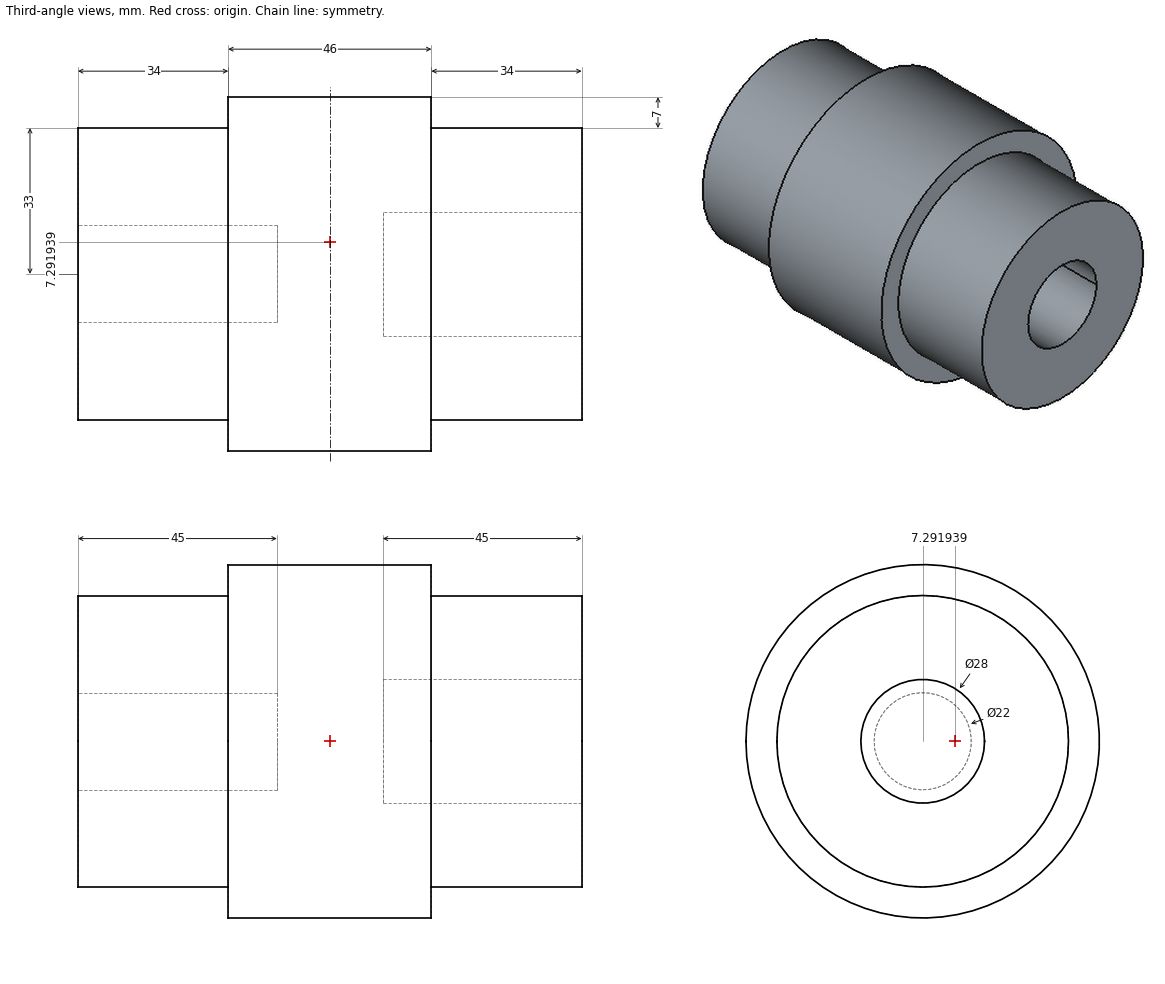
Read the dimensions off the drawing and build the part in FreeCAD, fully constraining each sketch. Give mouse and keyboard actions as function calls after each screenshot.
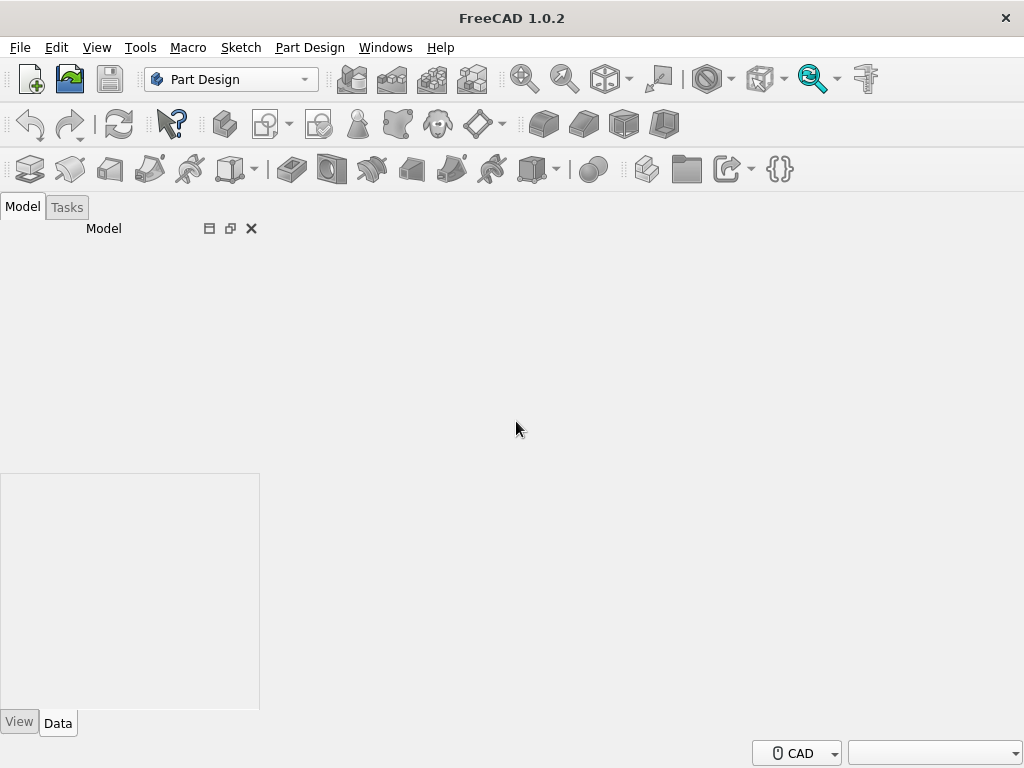
click(30, 80)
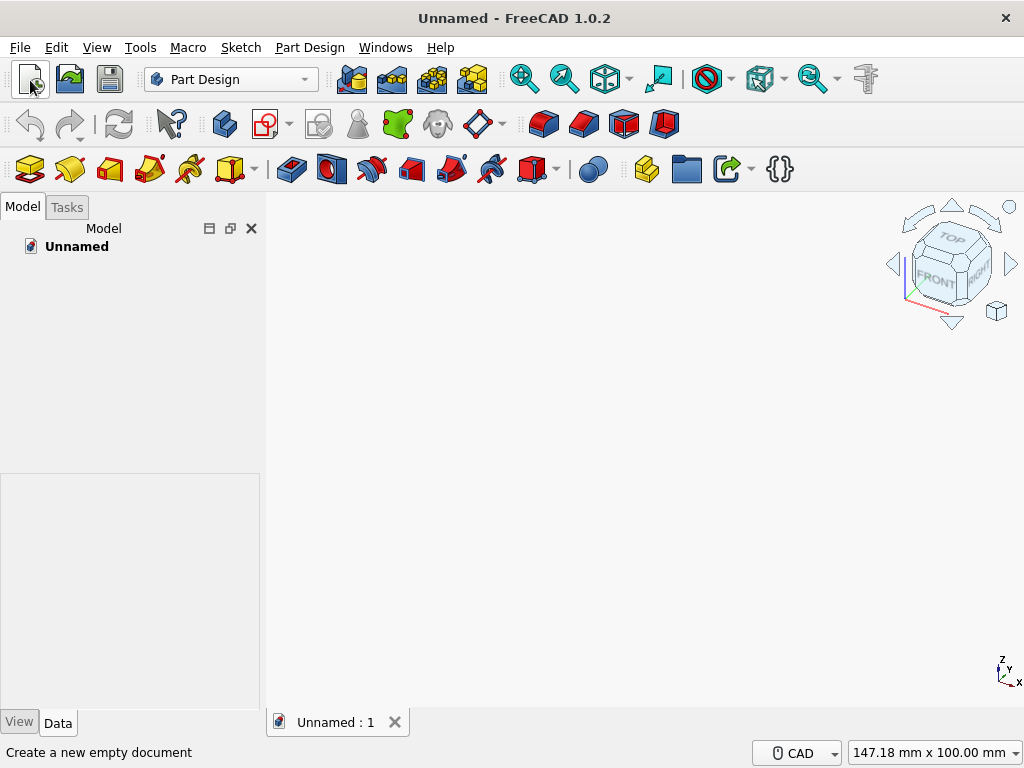
click(266, 124)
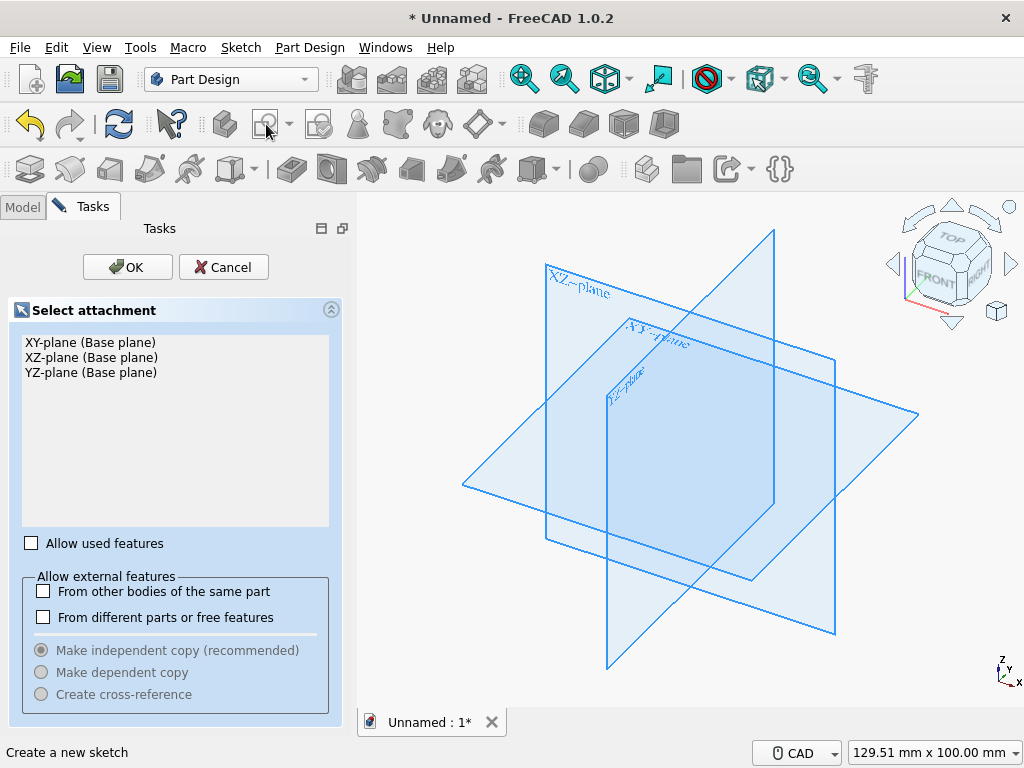
click(82, 342)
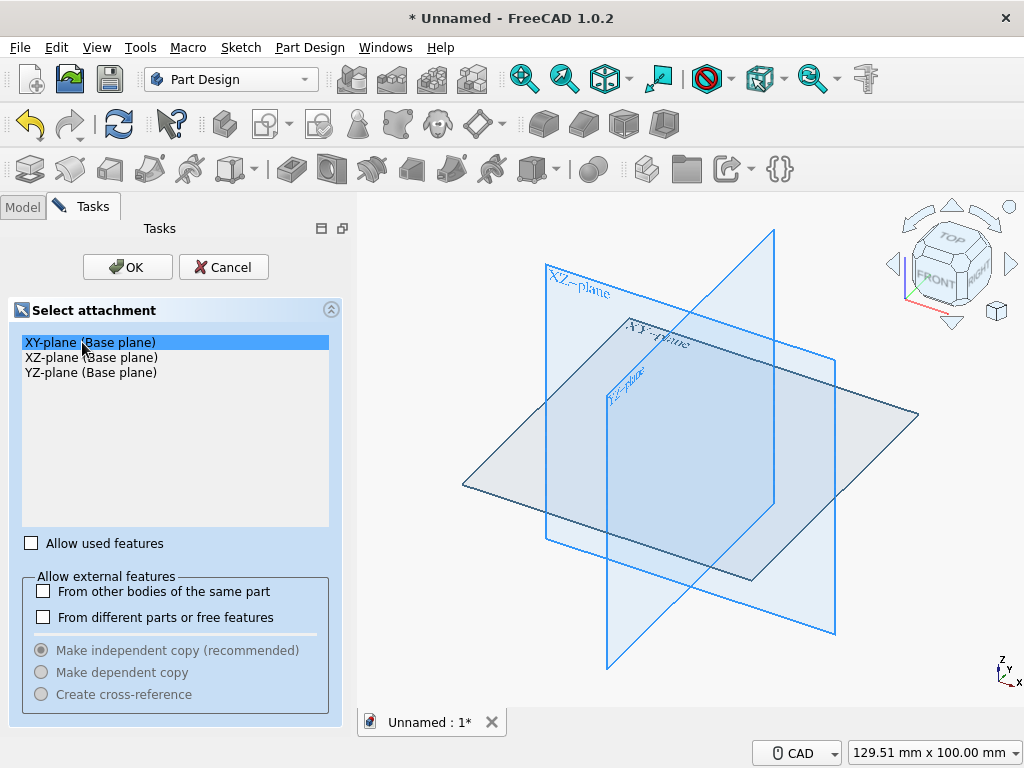
click(128, 267)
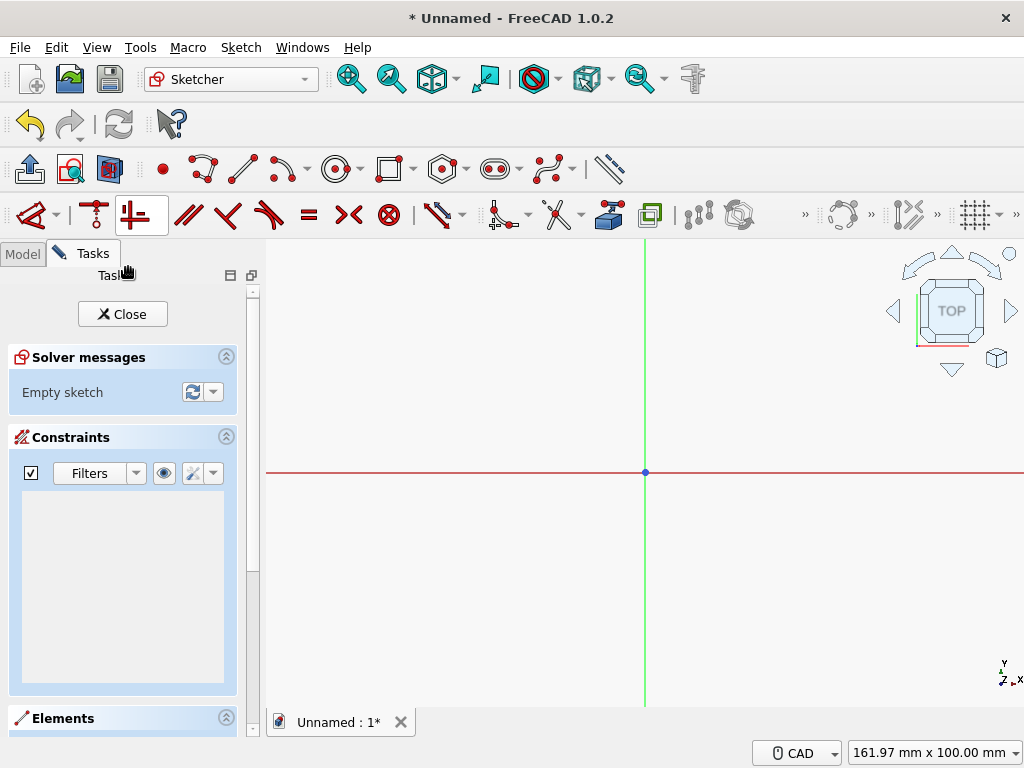
scroll(363, 545, down, 3)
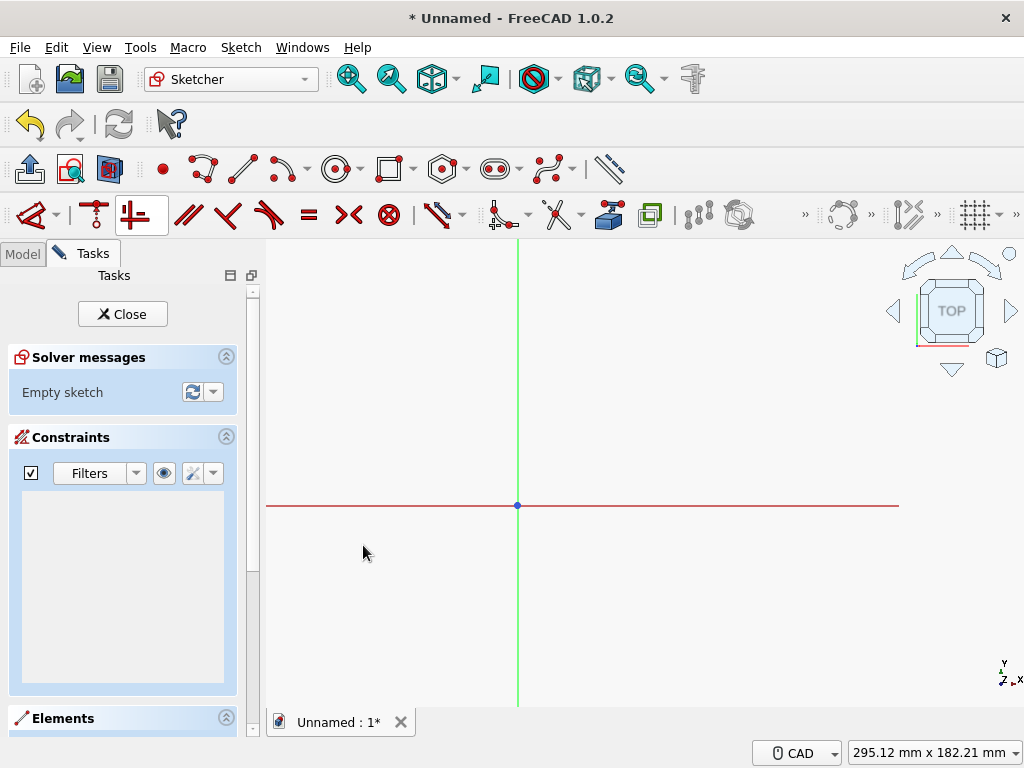
click(204, 170)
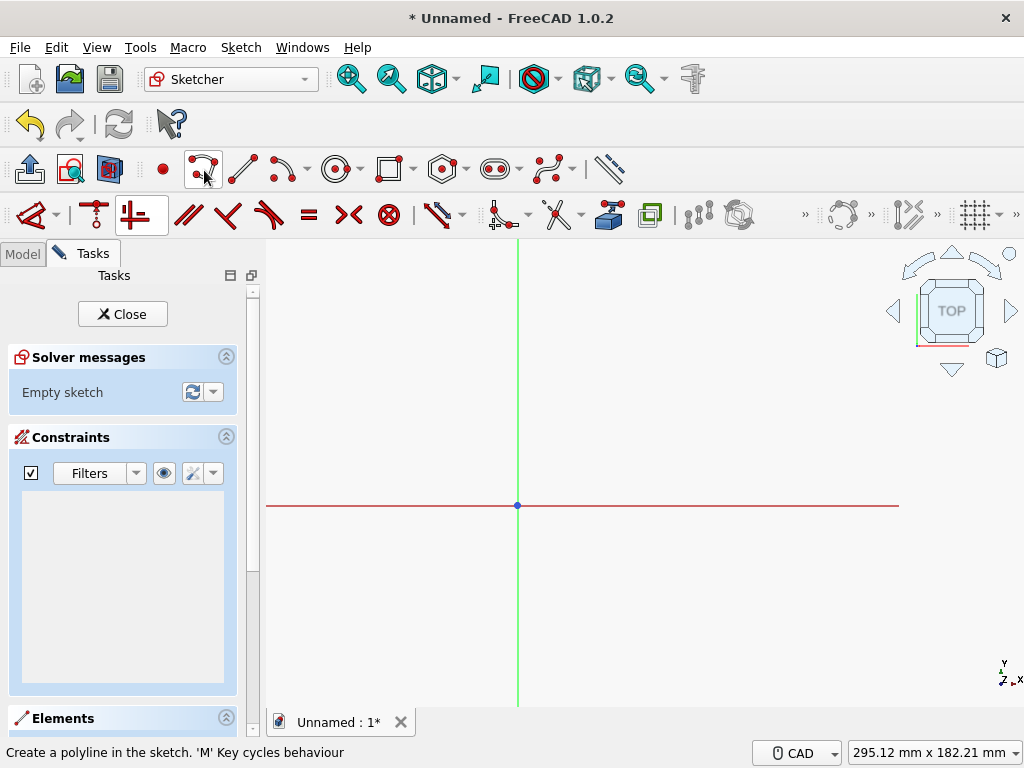
click(577, 440)
click(577, 422)
click(459, 422)
click(459, 440)
click(371, 440)
click(371, 525)
click(664, 525)
click(664, 440)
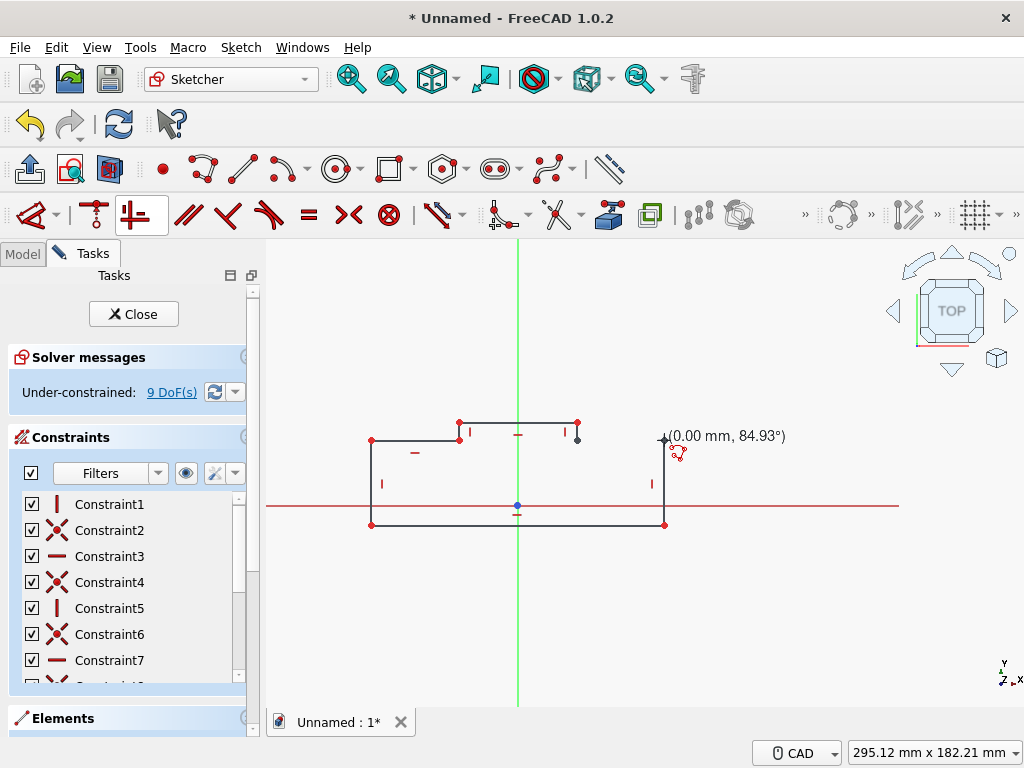
scroll(577, 440, up, 3)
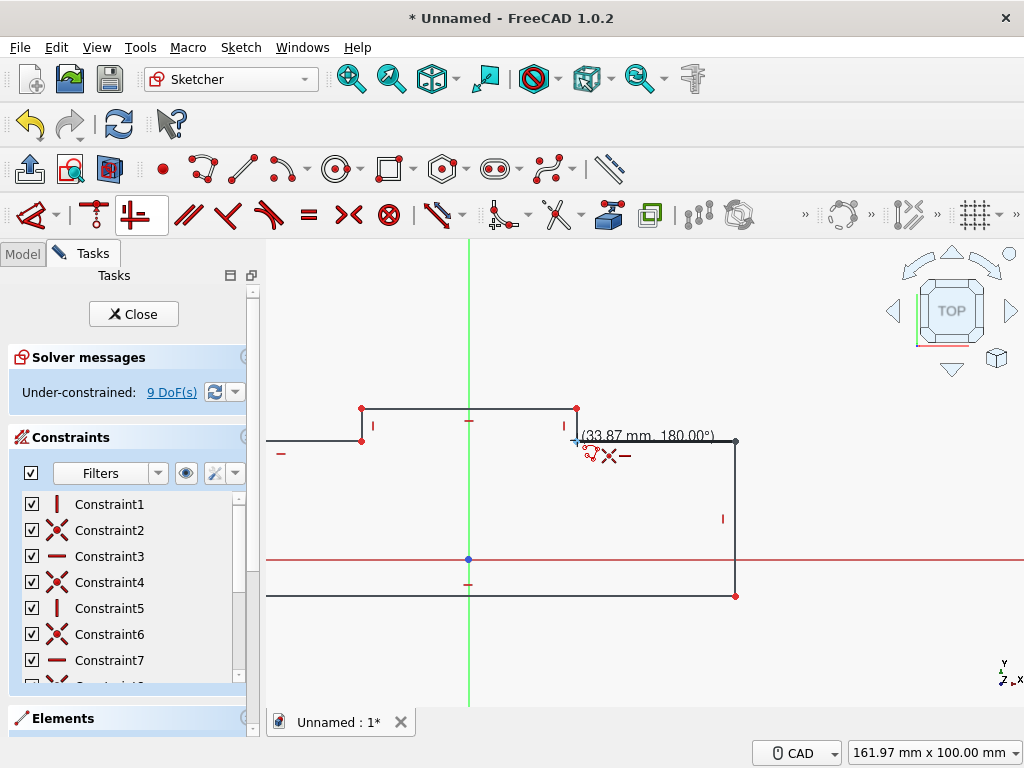
click(577, 441)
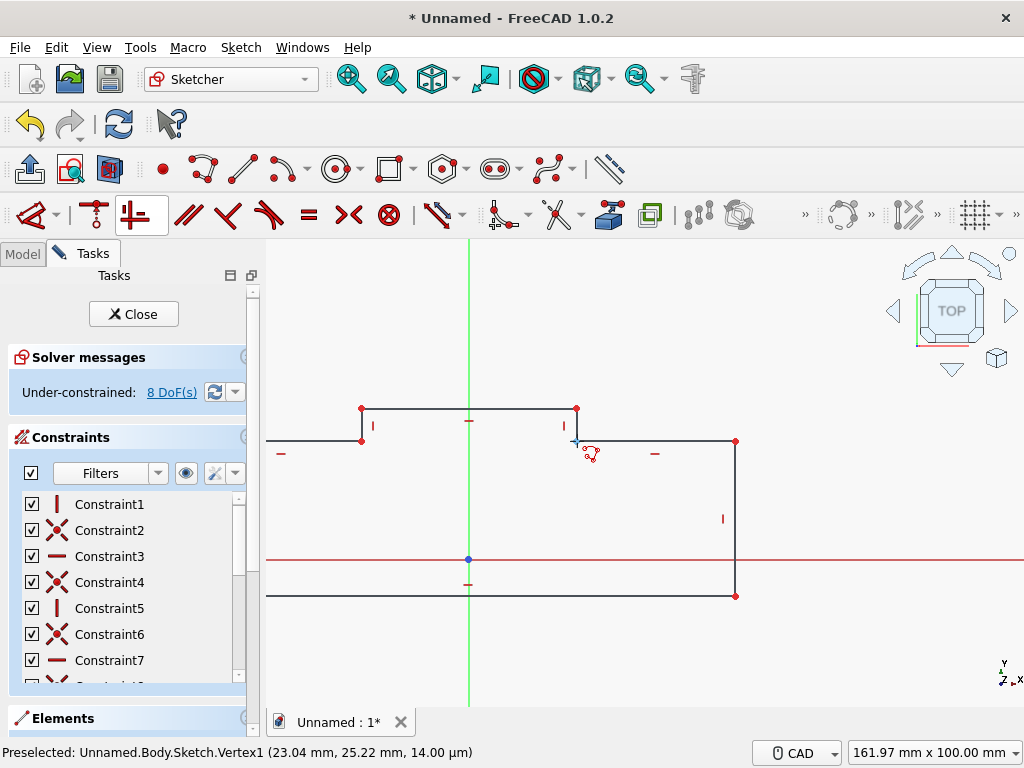
click(244, 170)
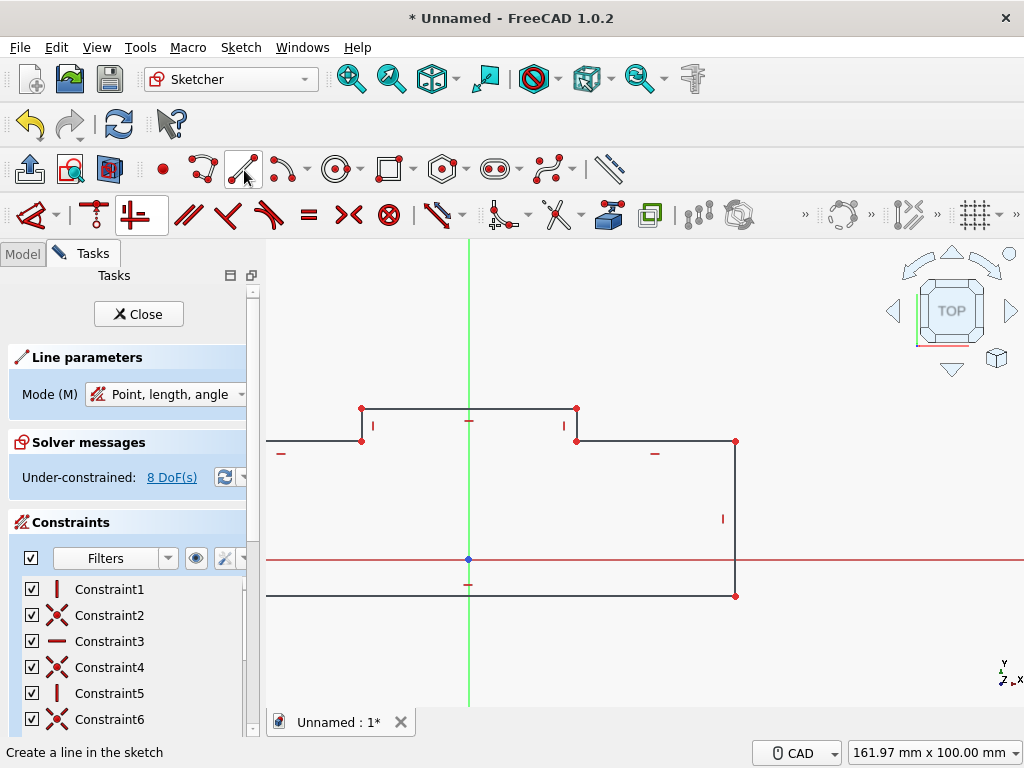
click(789, 594)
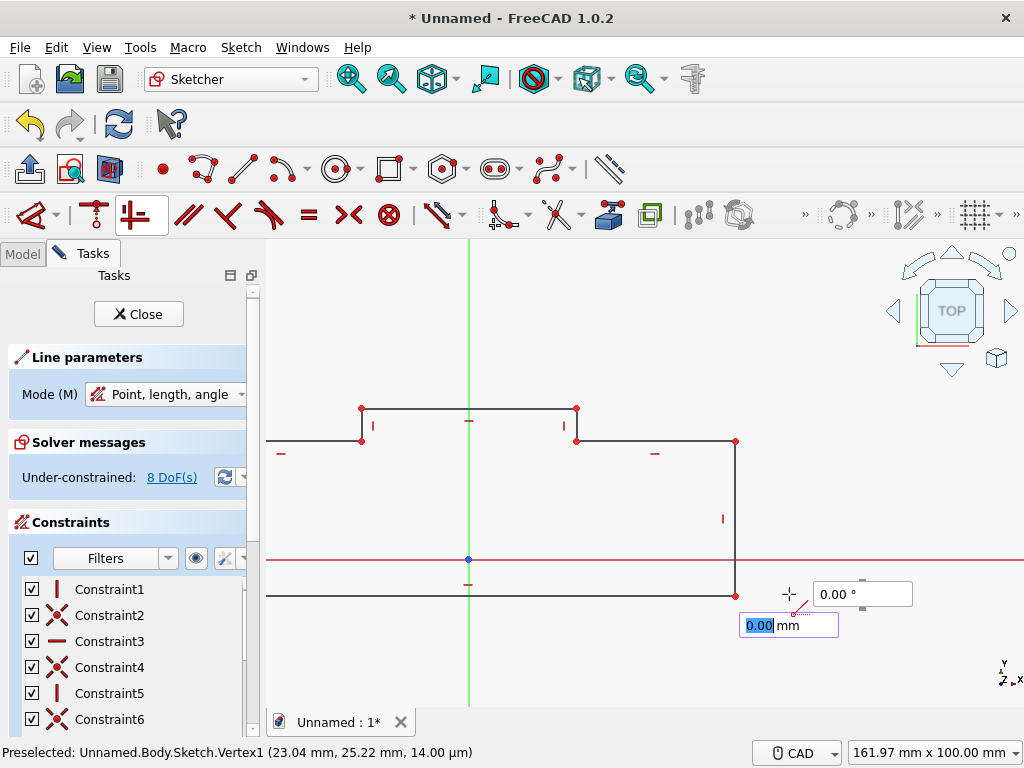
scroll(578, 440, down, 3)